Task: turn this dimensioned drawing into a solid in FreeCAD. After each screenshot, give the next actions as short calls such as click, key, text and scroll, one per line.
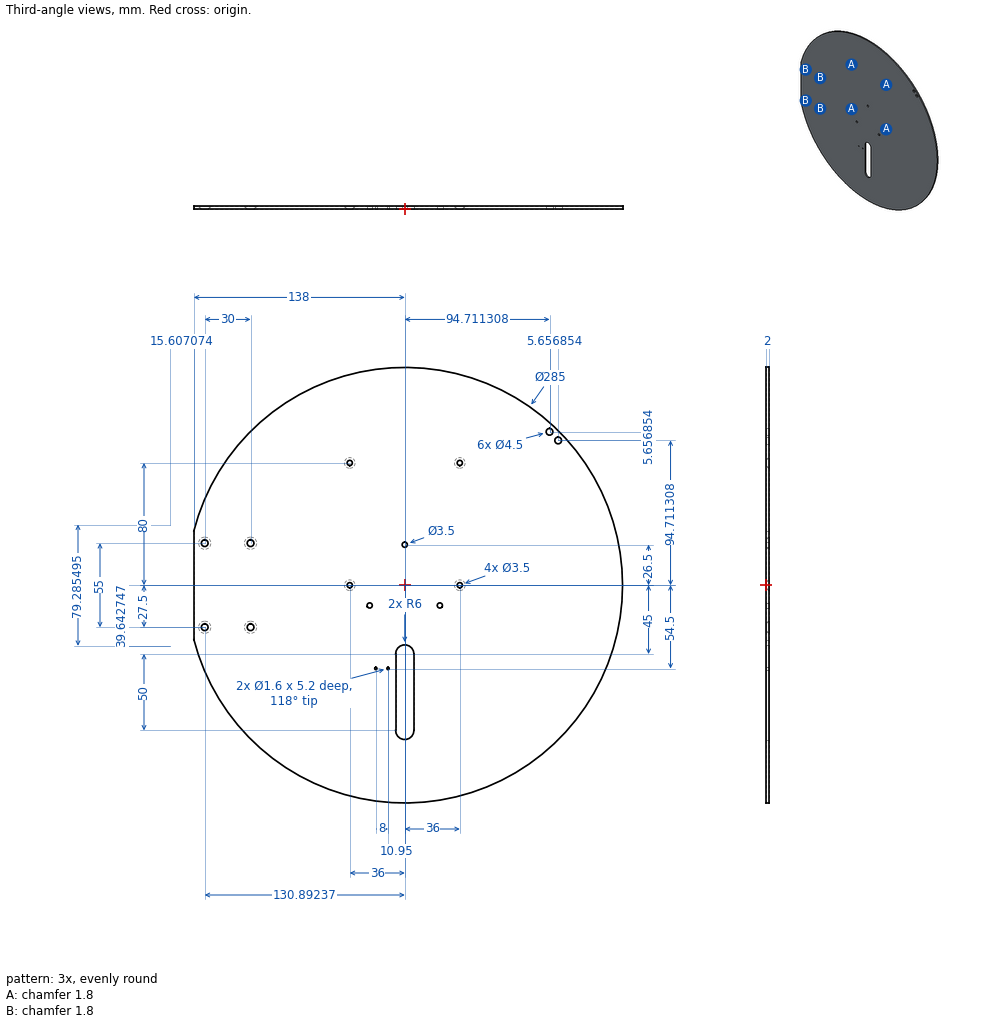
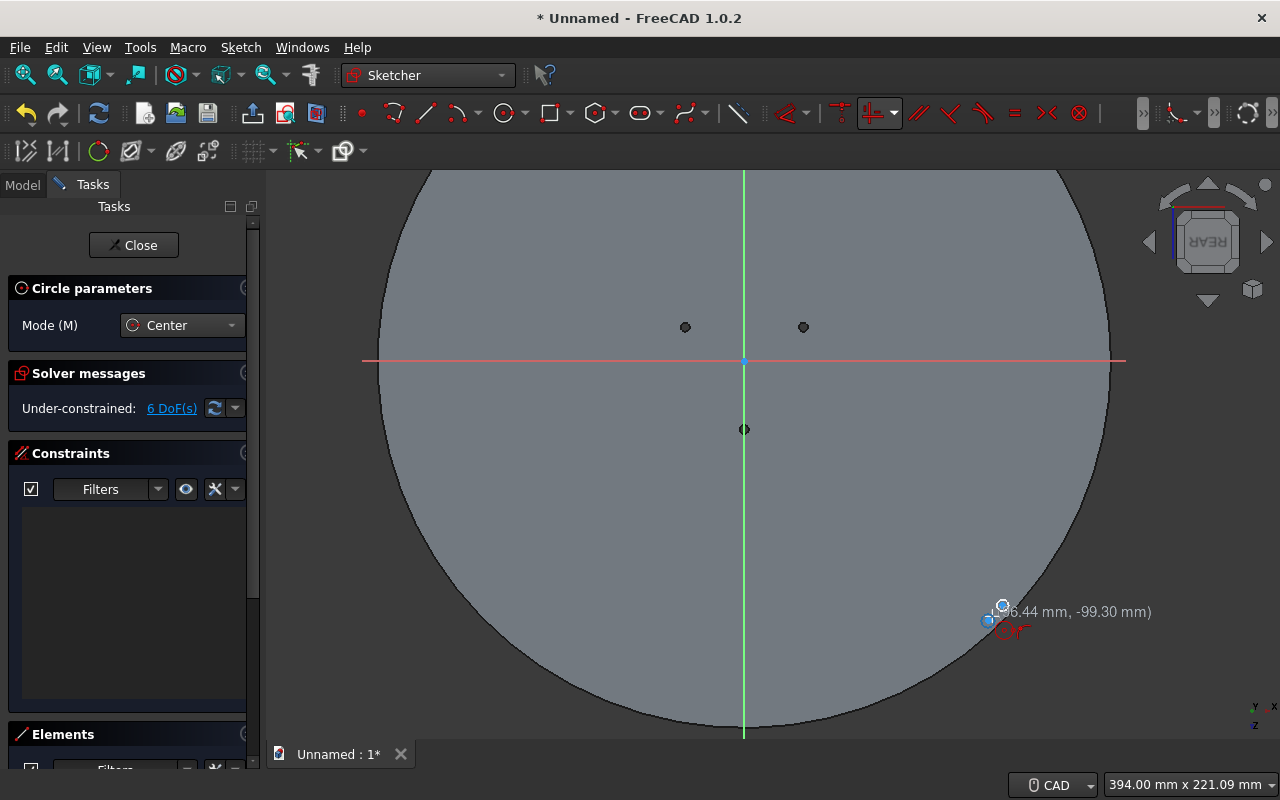
scroll(407, 291, up, 7)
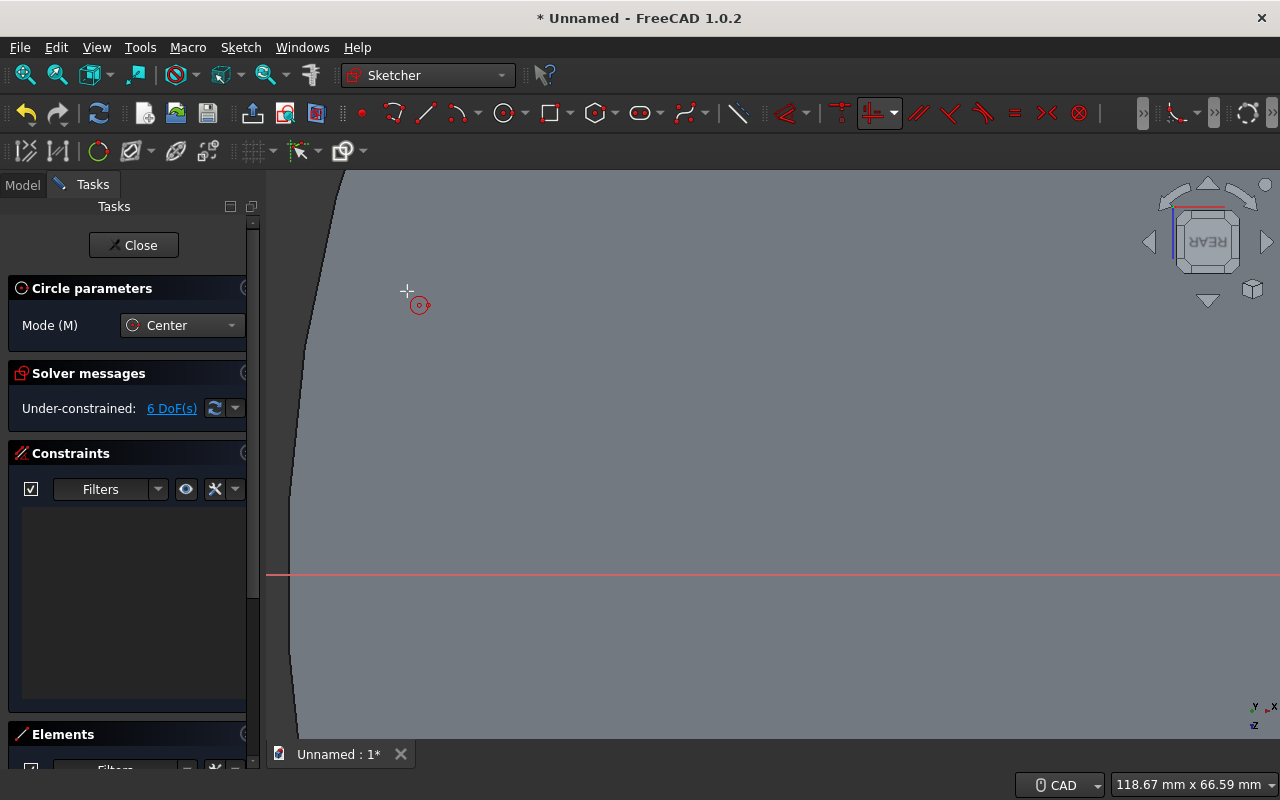
scroll(406, 290, down, 7)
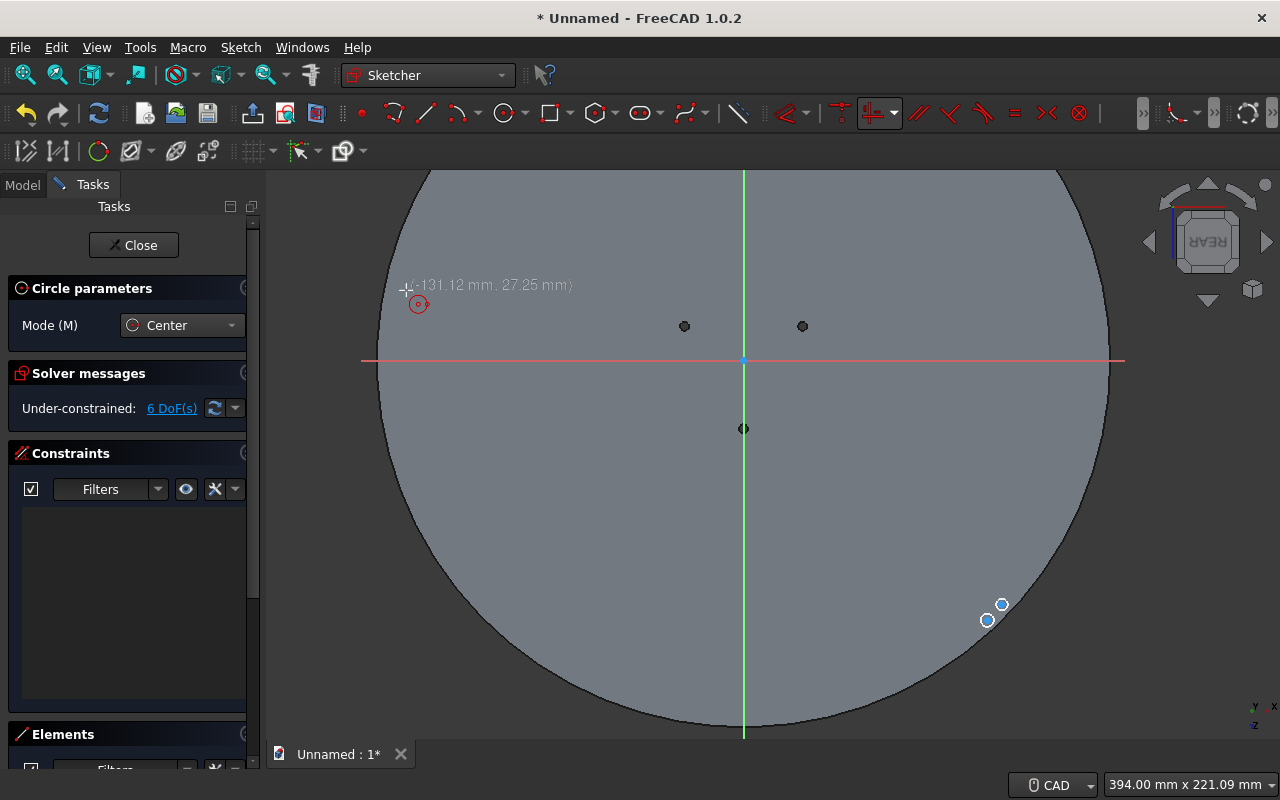
click(407, 290)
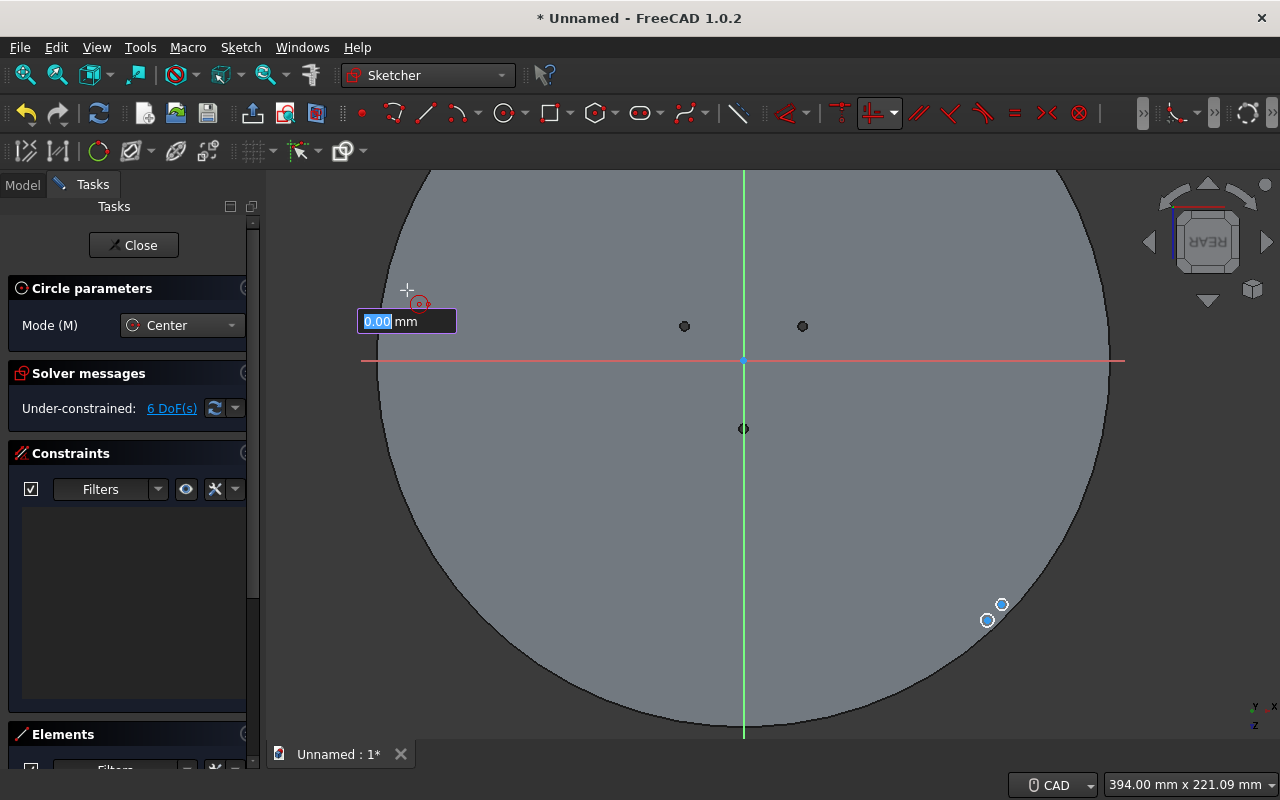
scroll(411, 286, up, 6)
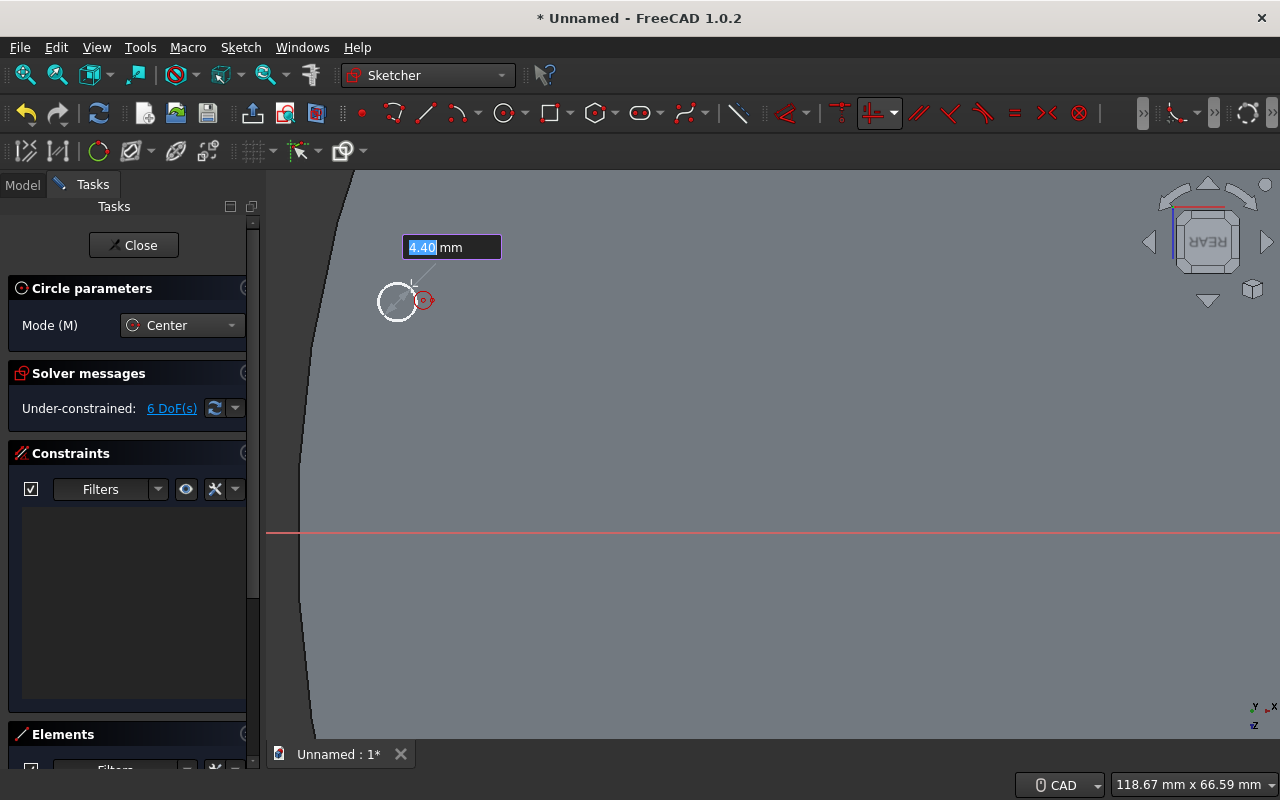
click(410, 284)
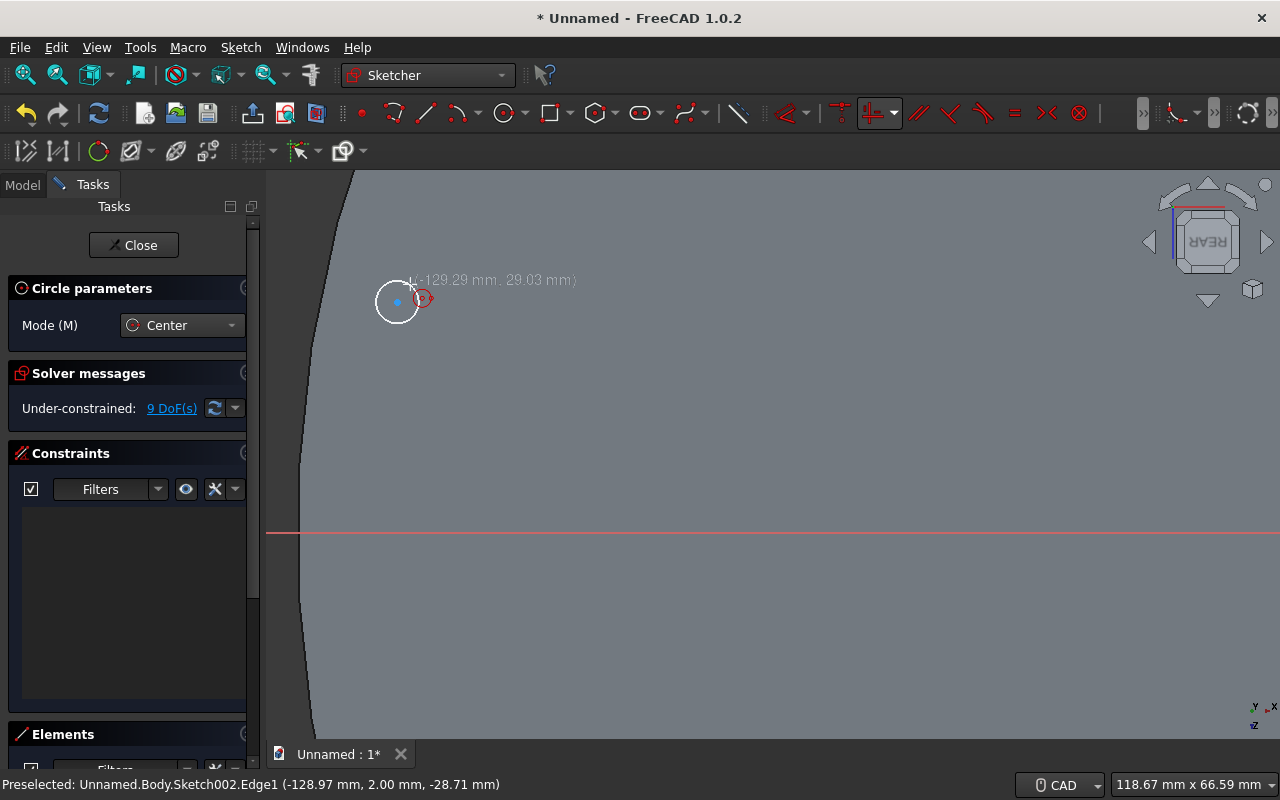
scroll(411, 286, down, 6)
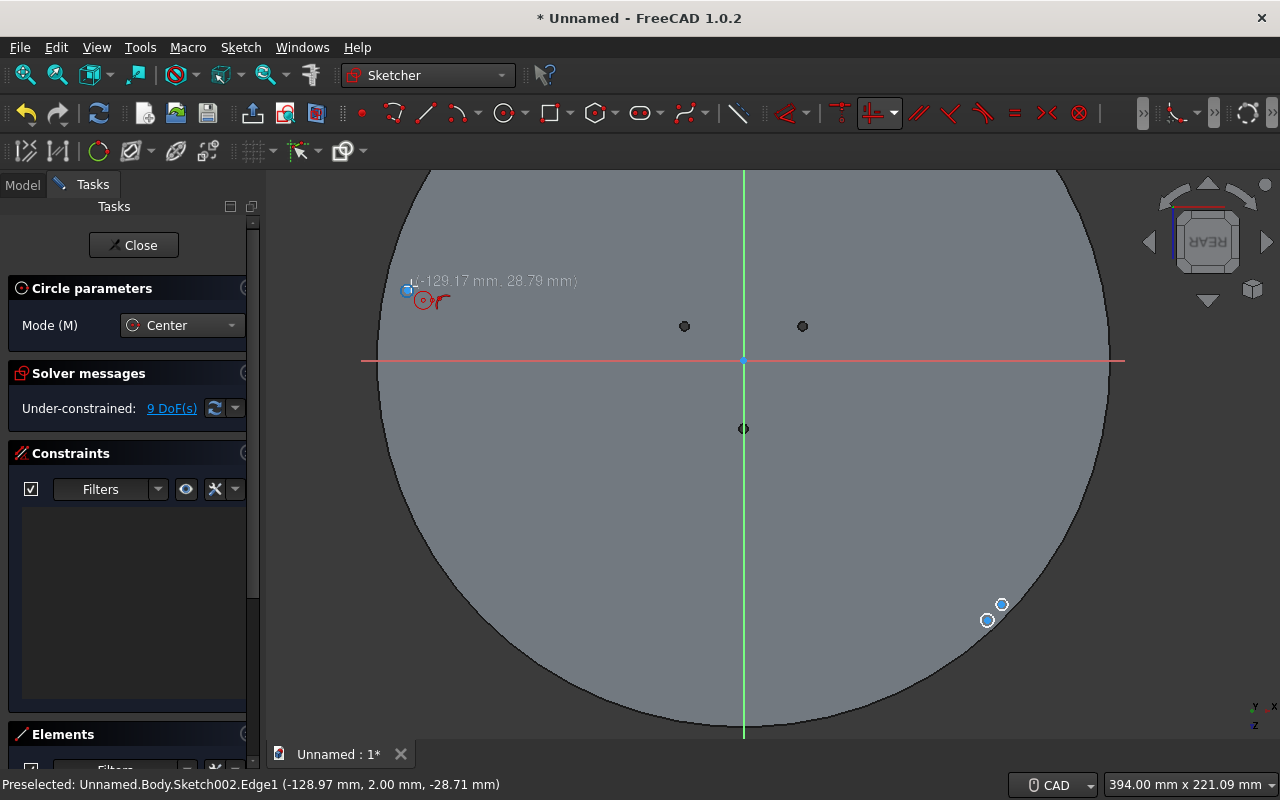
scroll(407, 431, up, 7)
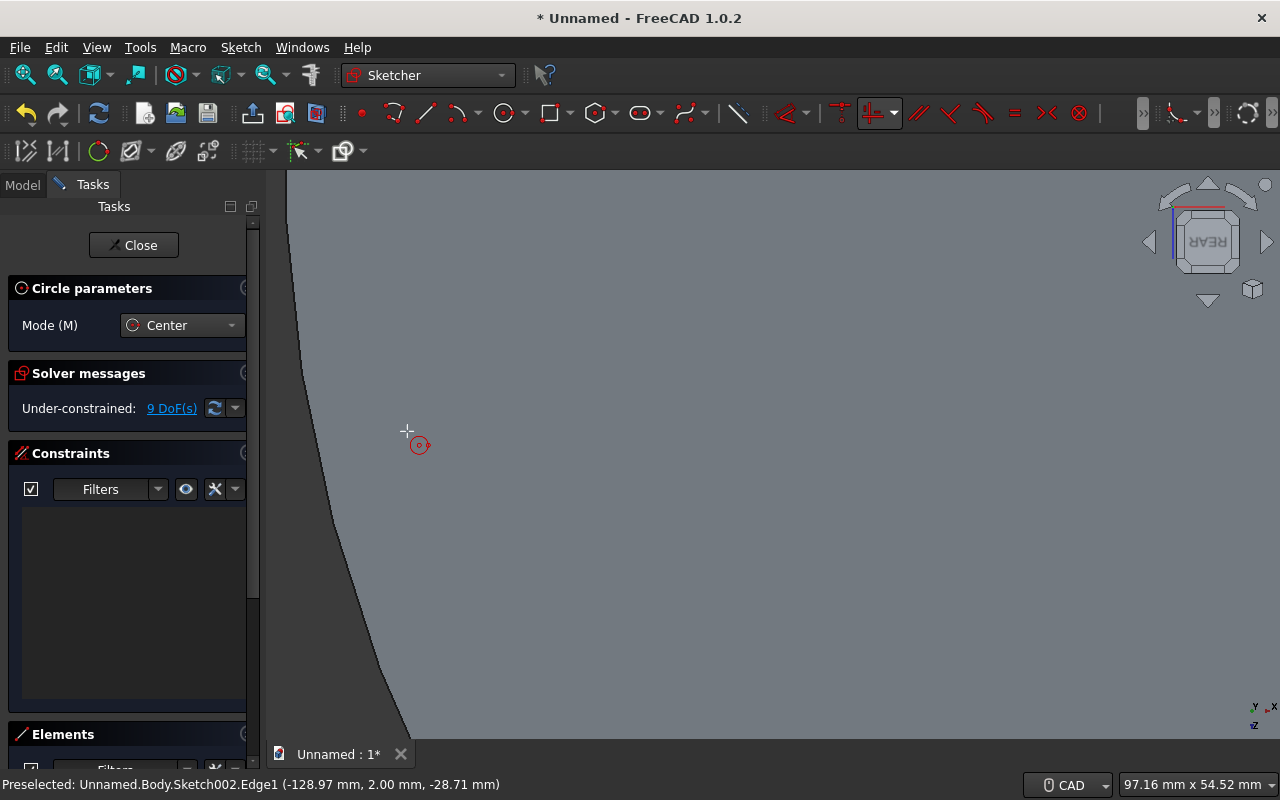
scroll(407, 432, down, 7)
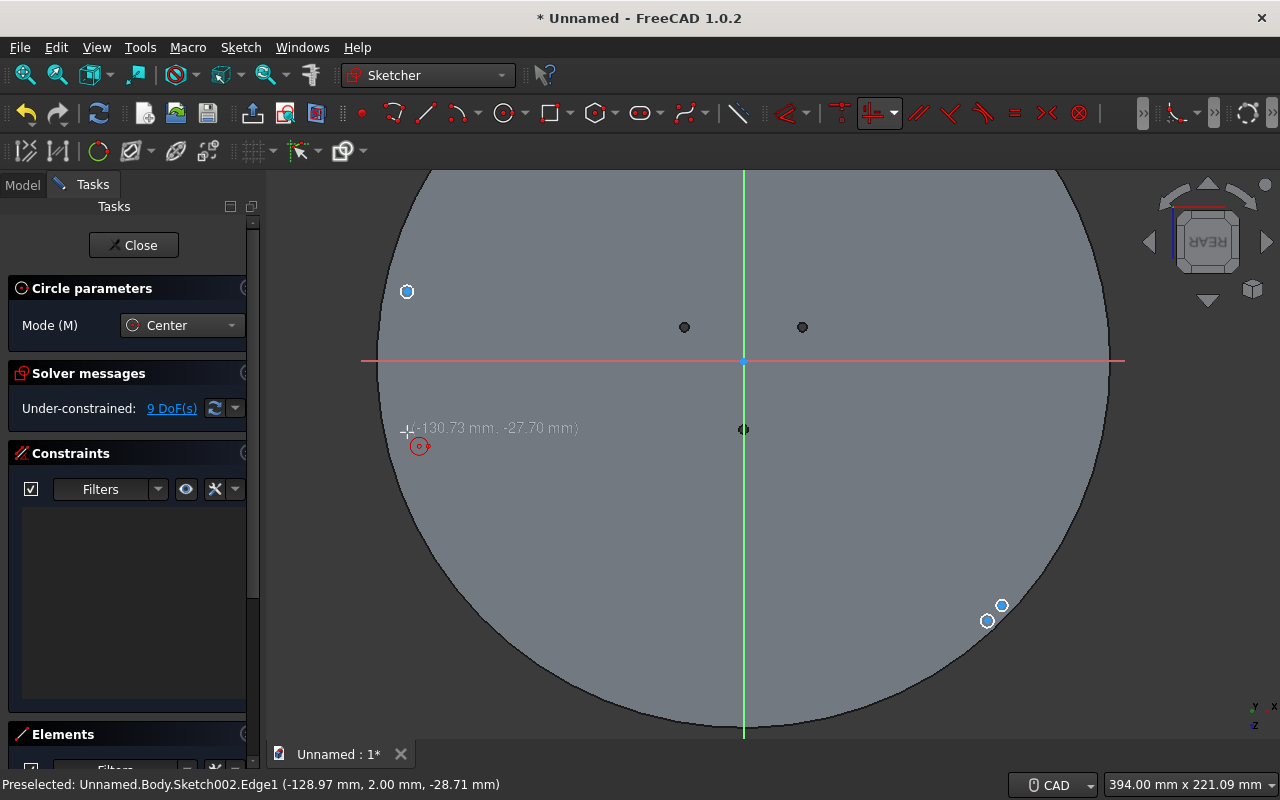
click(407, 432)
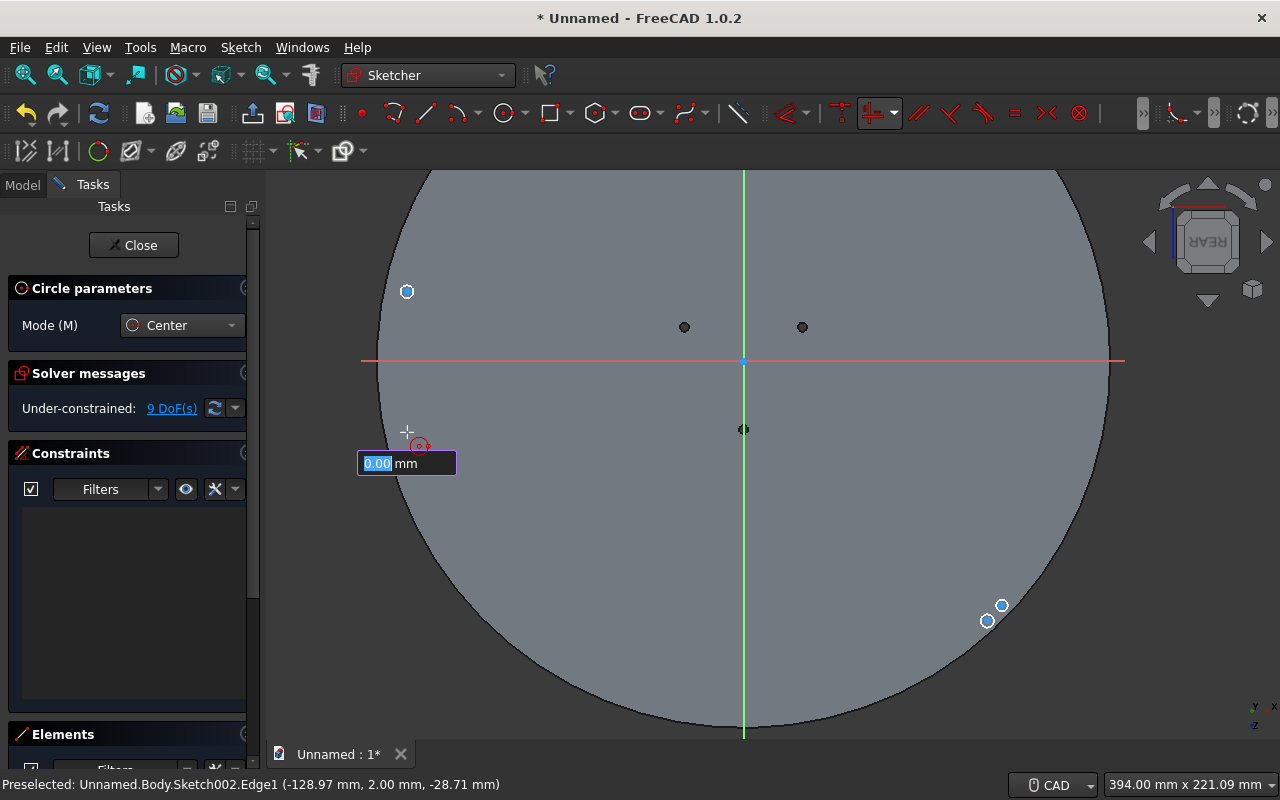
scroll(411, 428, up, 6)